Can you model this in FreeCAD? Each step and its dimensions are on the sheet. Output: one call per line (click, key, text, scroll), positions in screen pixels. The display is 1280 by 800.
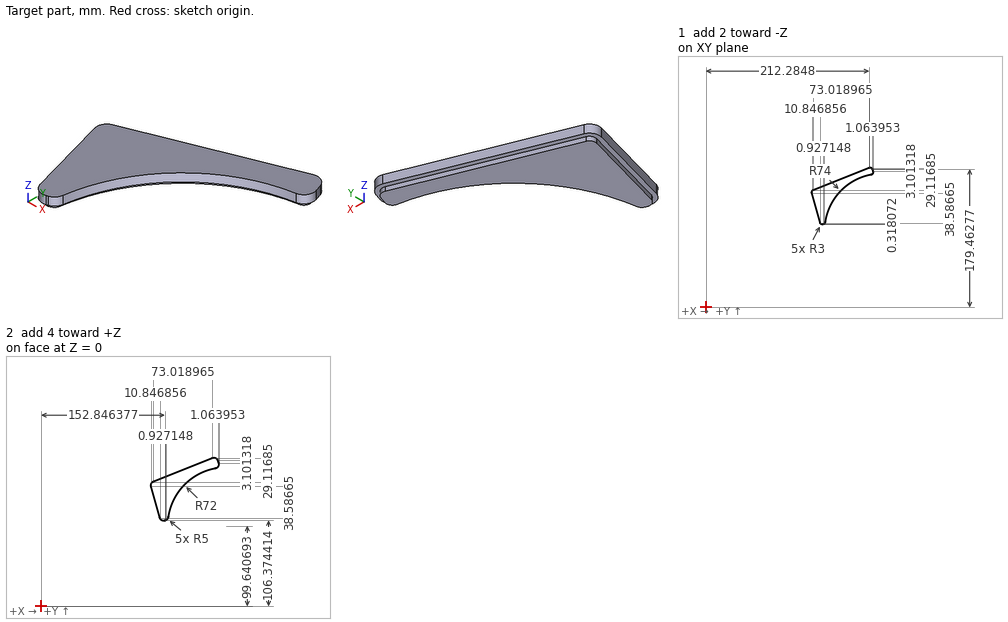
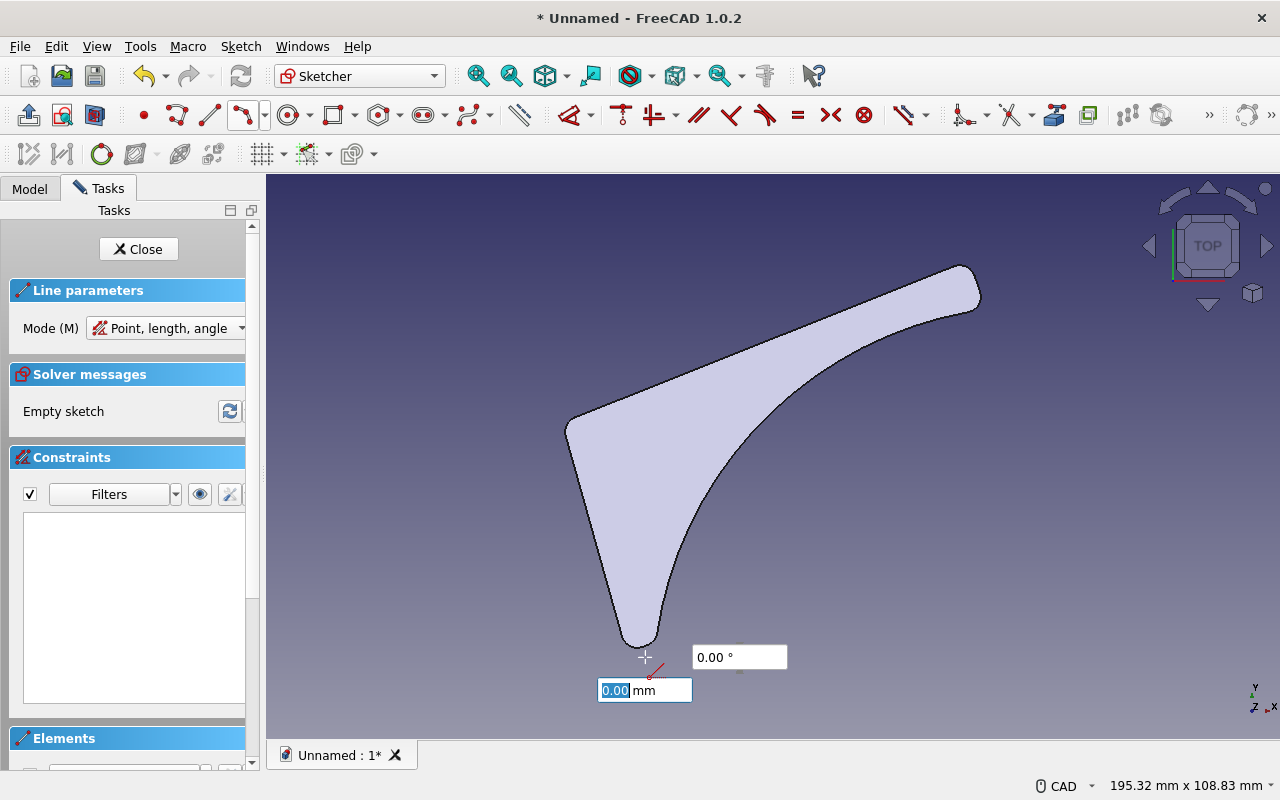
scroll(650, 655, up, 6)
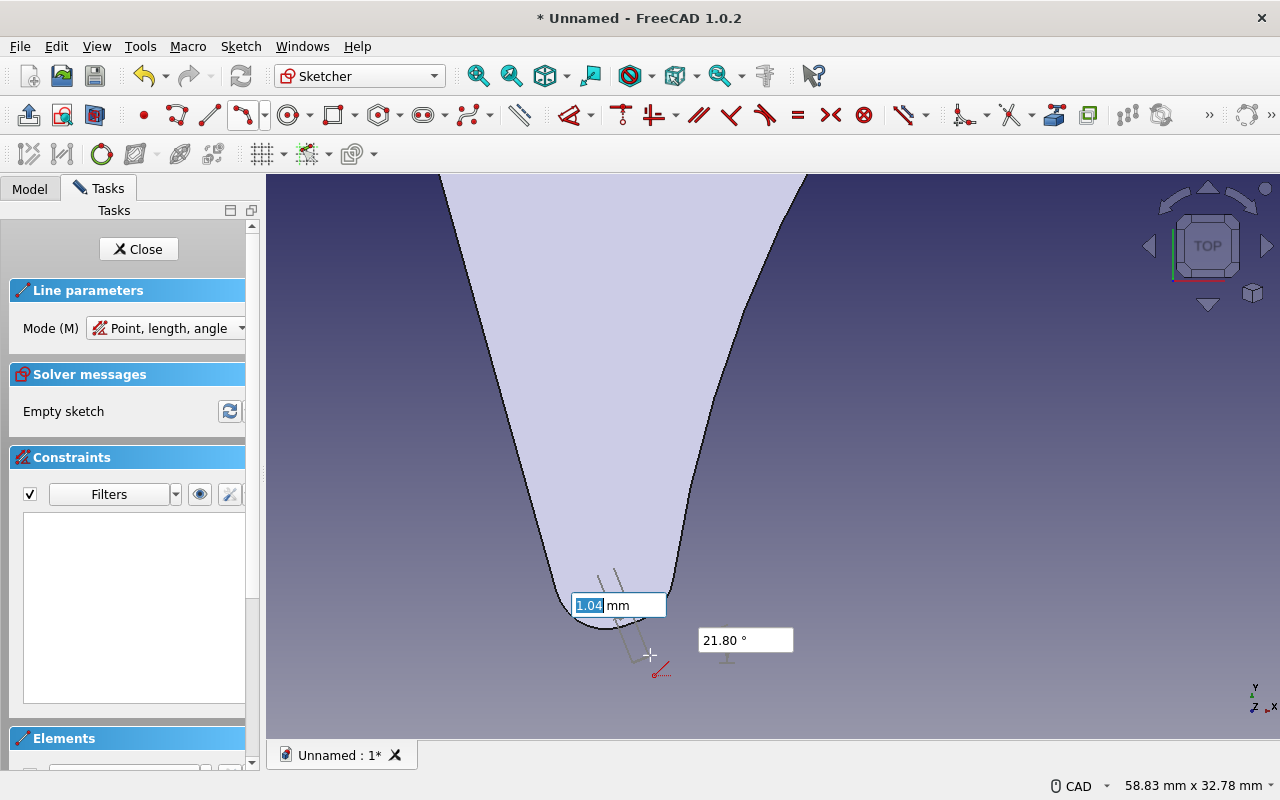
click(650, 654)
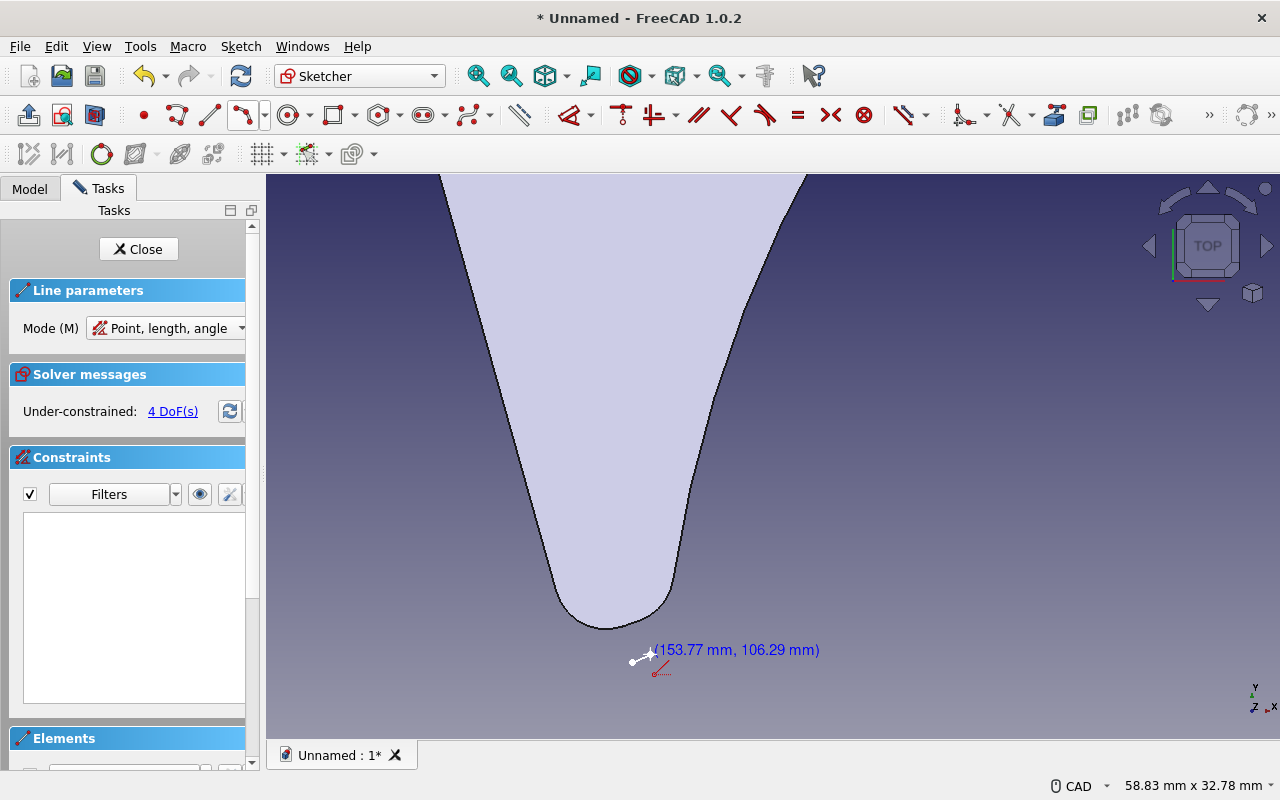
scroll(589, 608, down, 7)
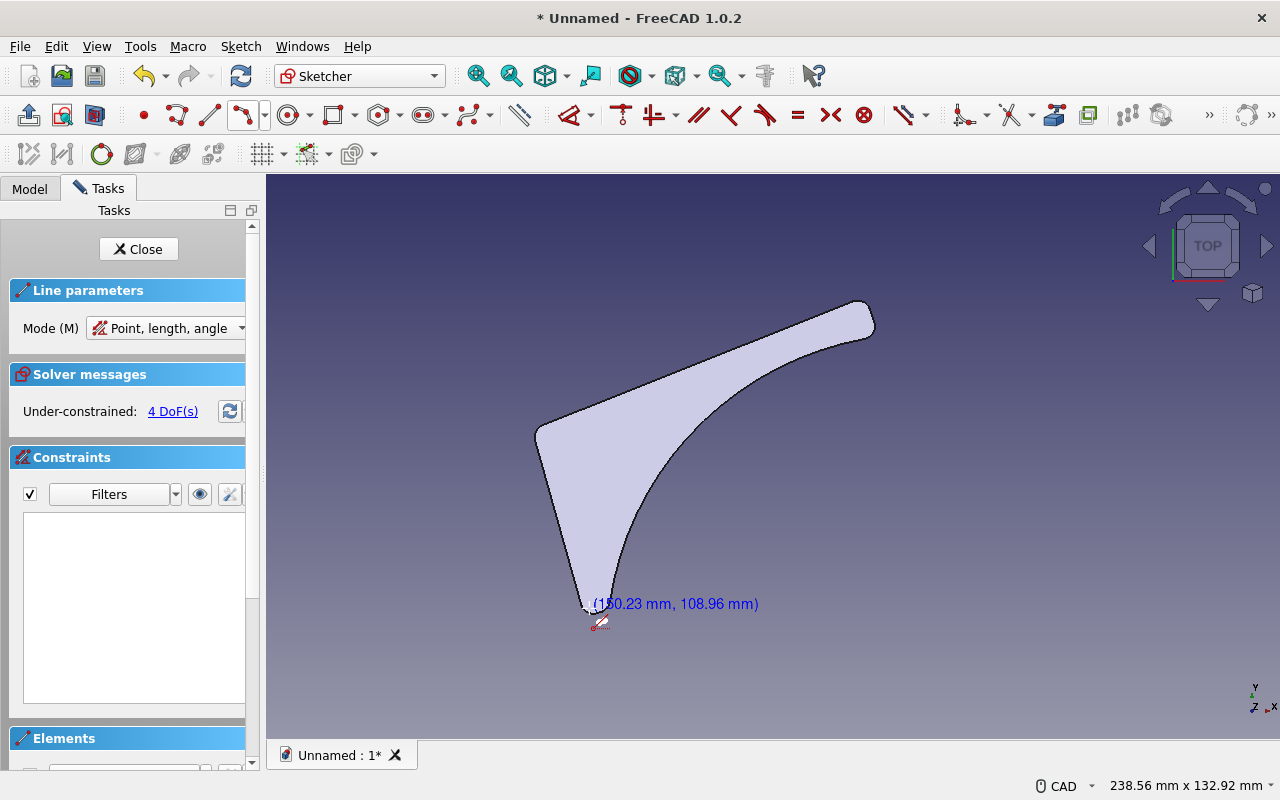
click(882, 320)
click(878, 306)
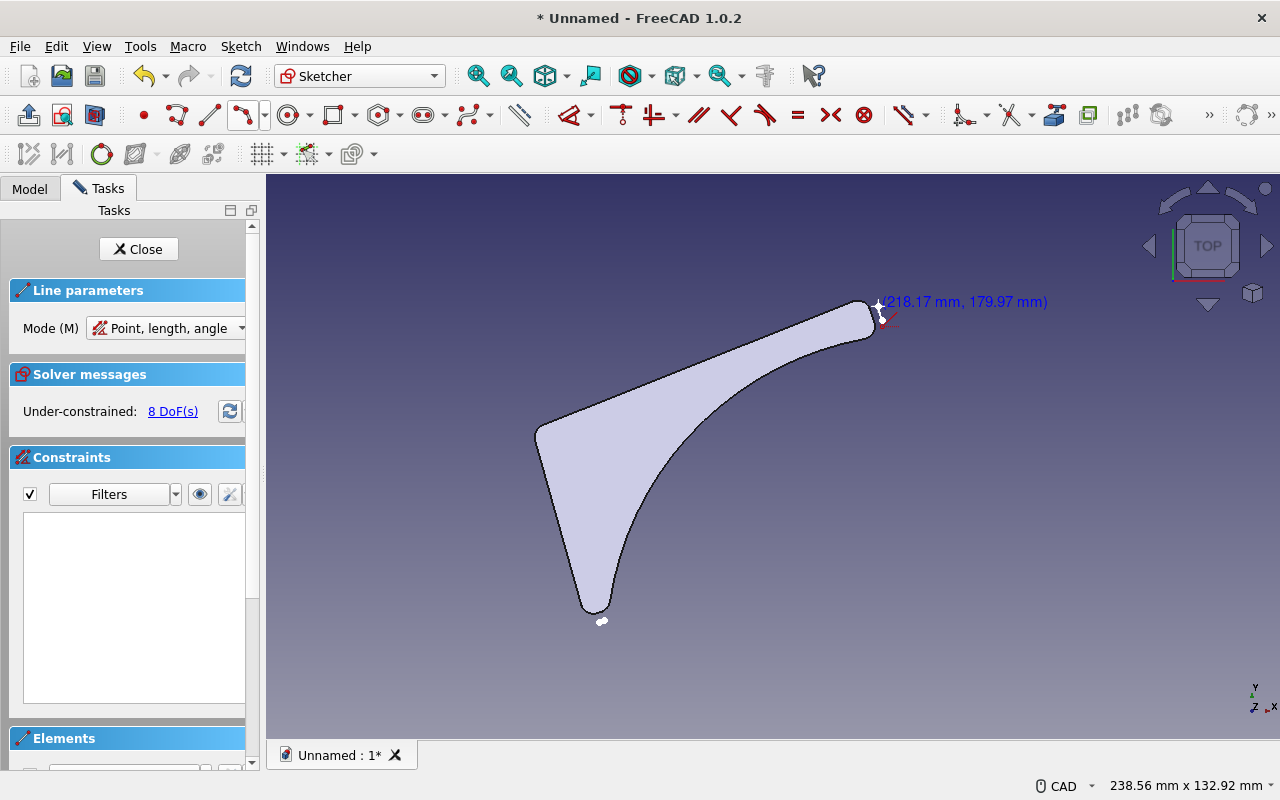
click(850, 294)
click(539, 417)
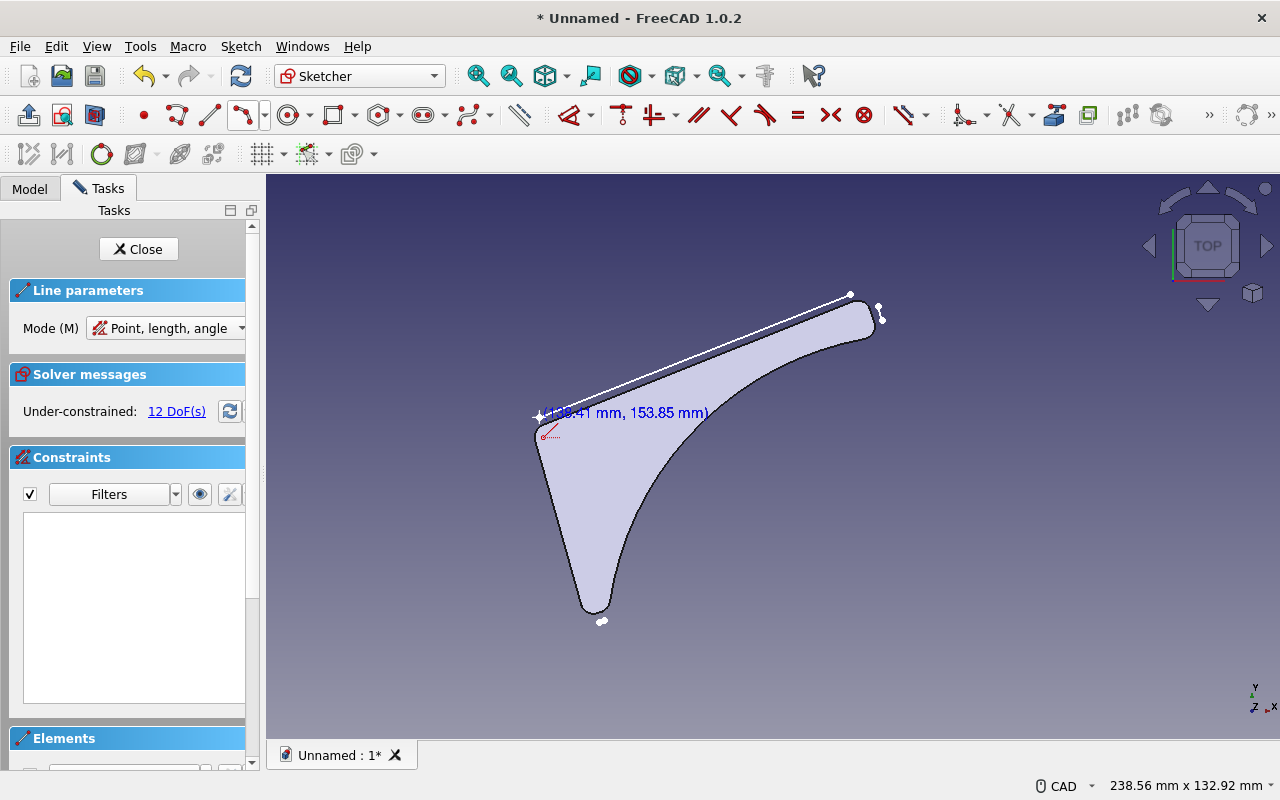
click(527, 443)
click(573, 607)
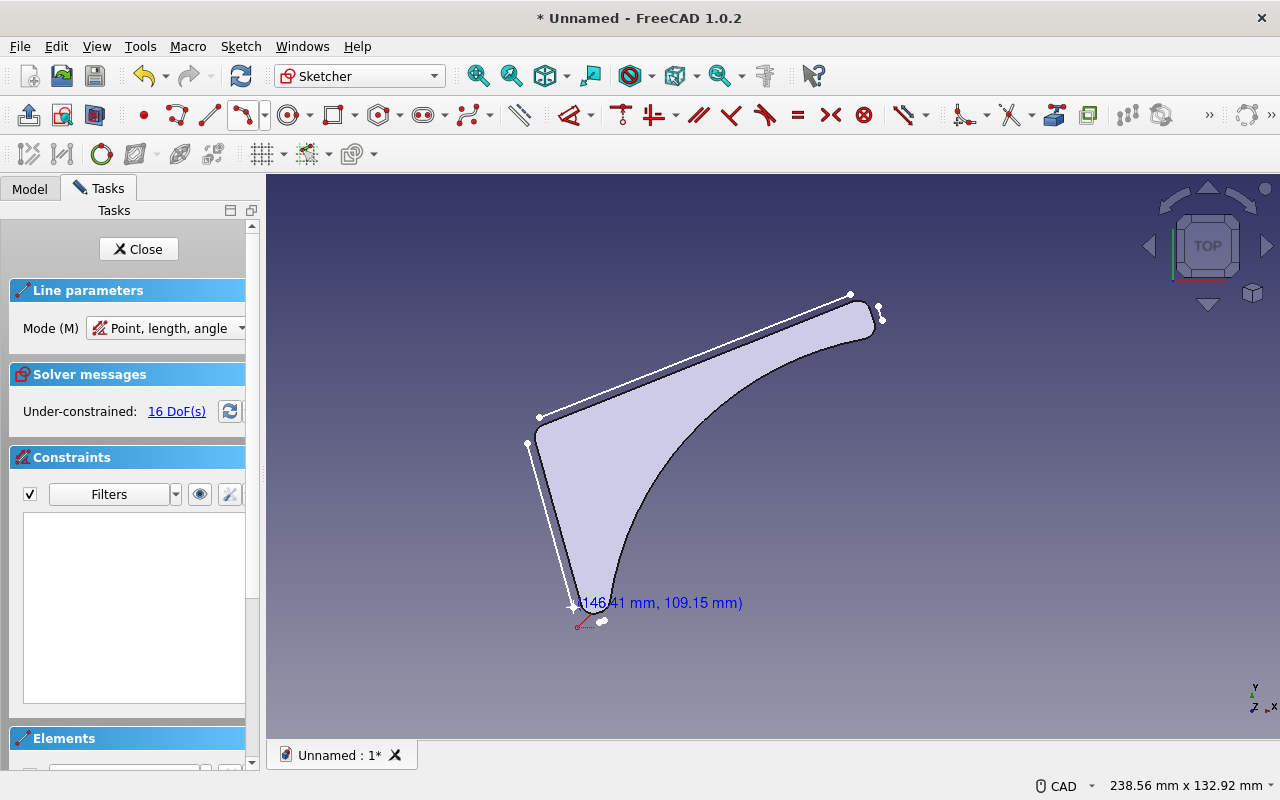
click(242, 116)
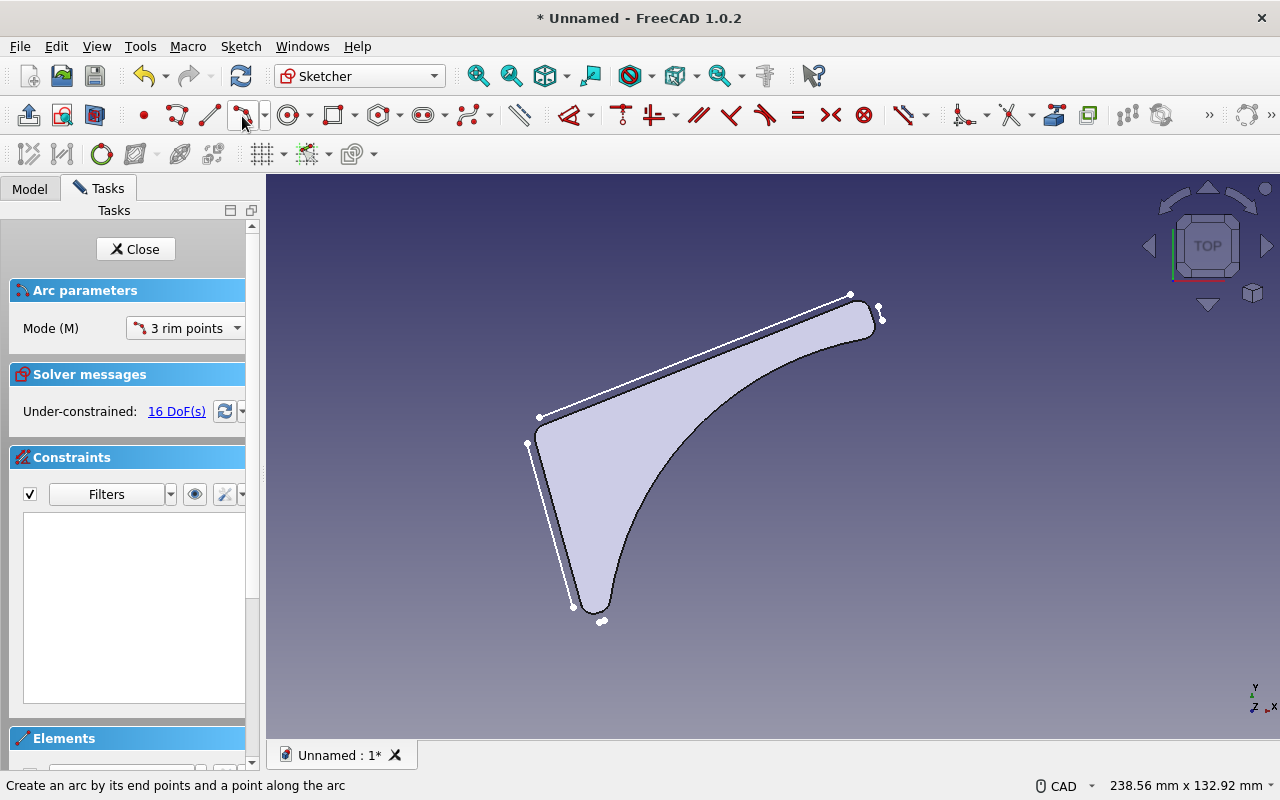
scroll(604, 620, up, 11)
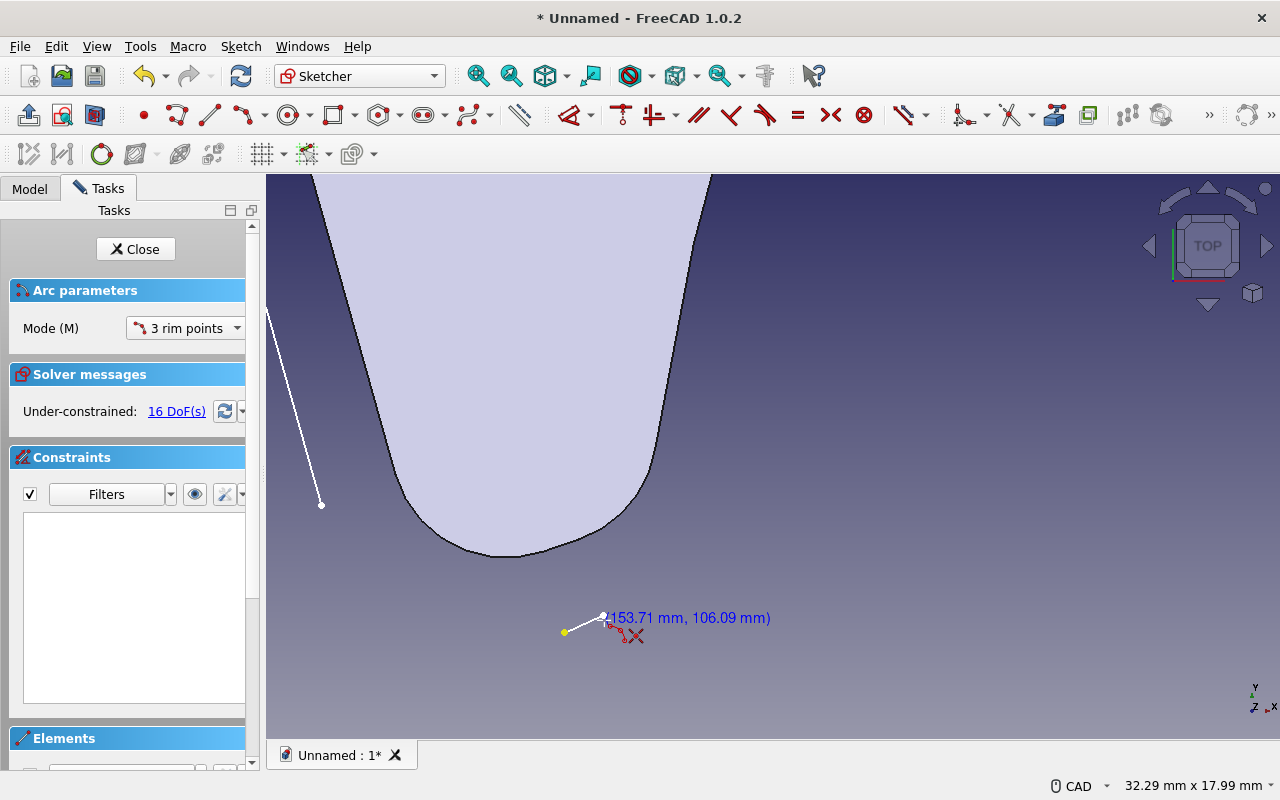
click(604, 615)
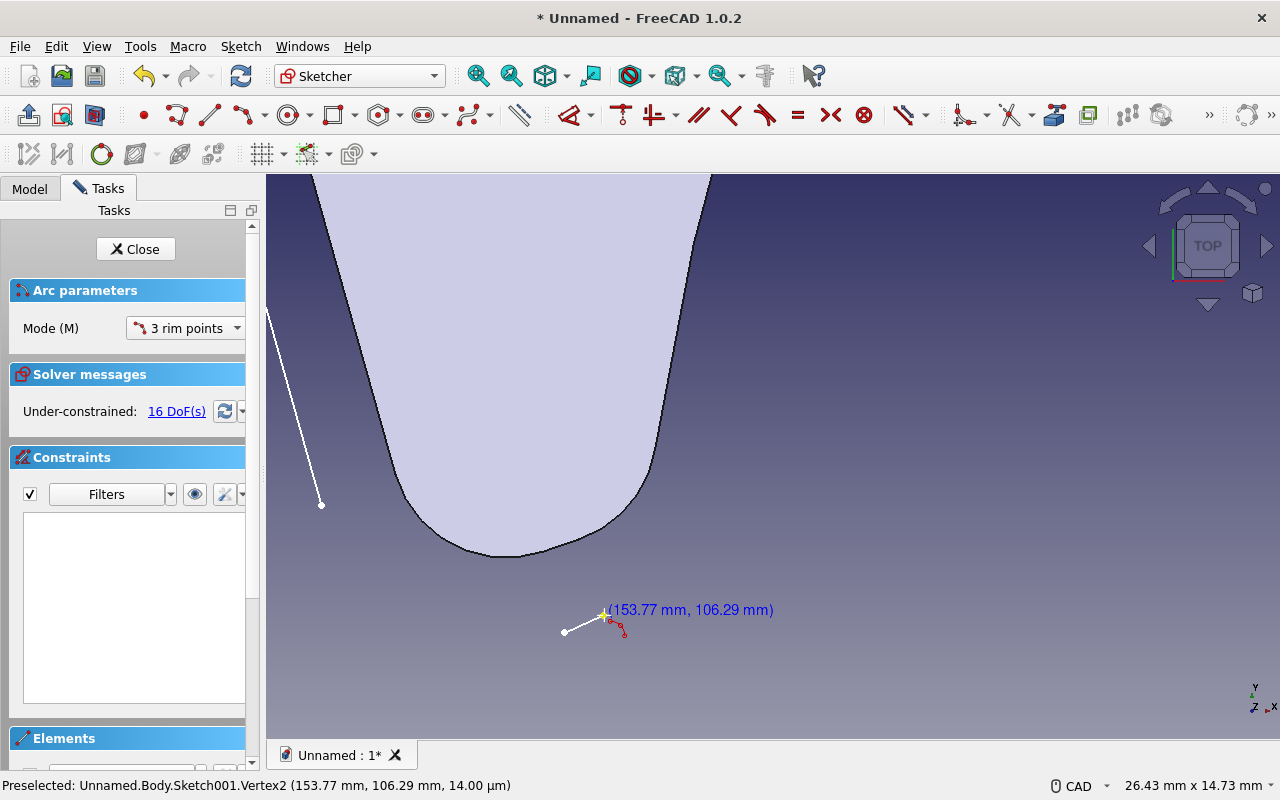
scroll(604, 620, down, 11)